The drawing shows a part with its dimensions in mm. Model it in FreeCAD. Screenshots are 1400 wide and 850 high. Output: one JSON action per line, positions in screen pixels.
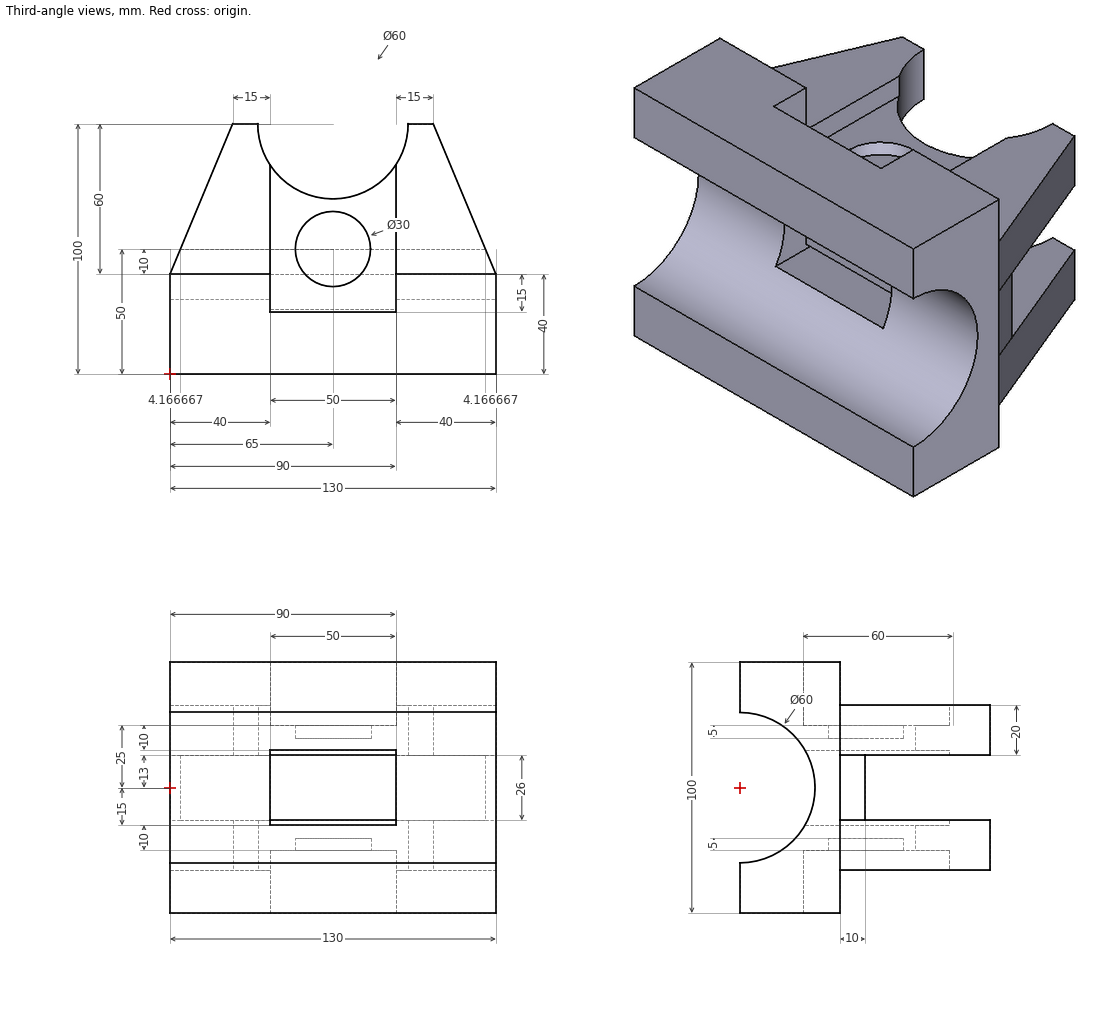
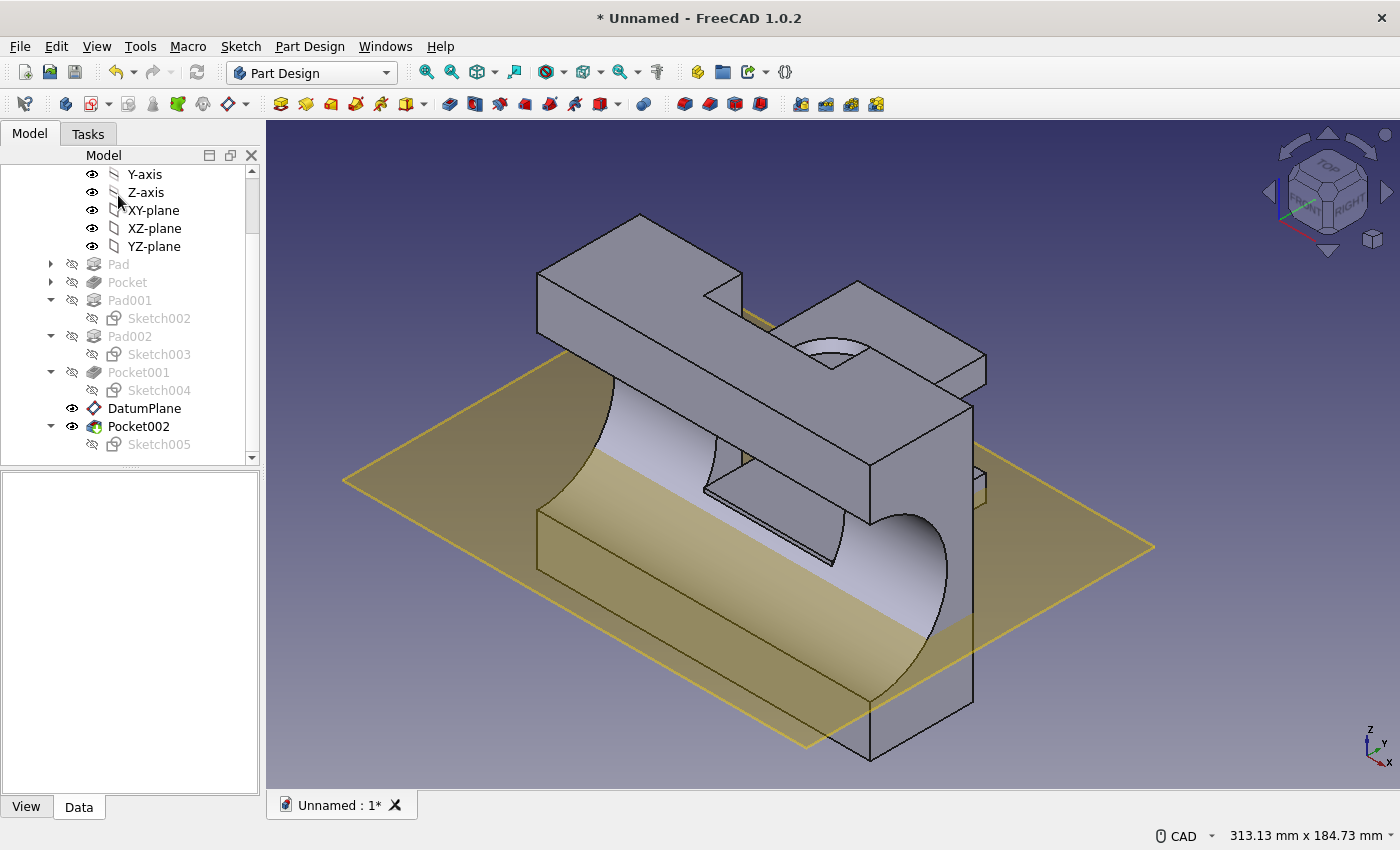
{"action": "left_click", "coordinate": [117, 408]}
{"action": "key", "text": "space"}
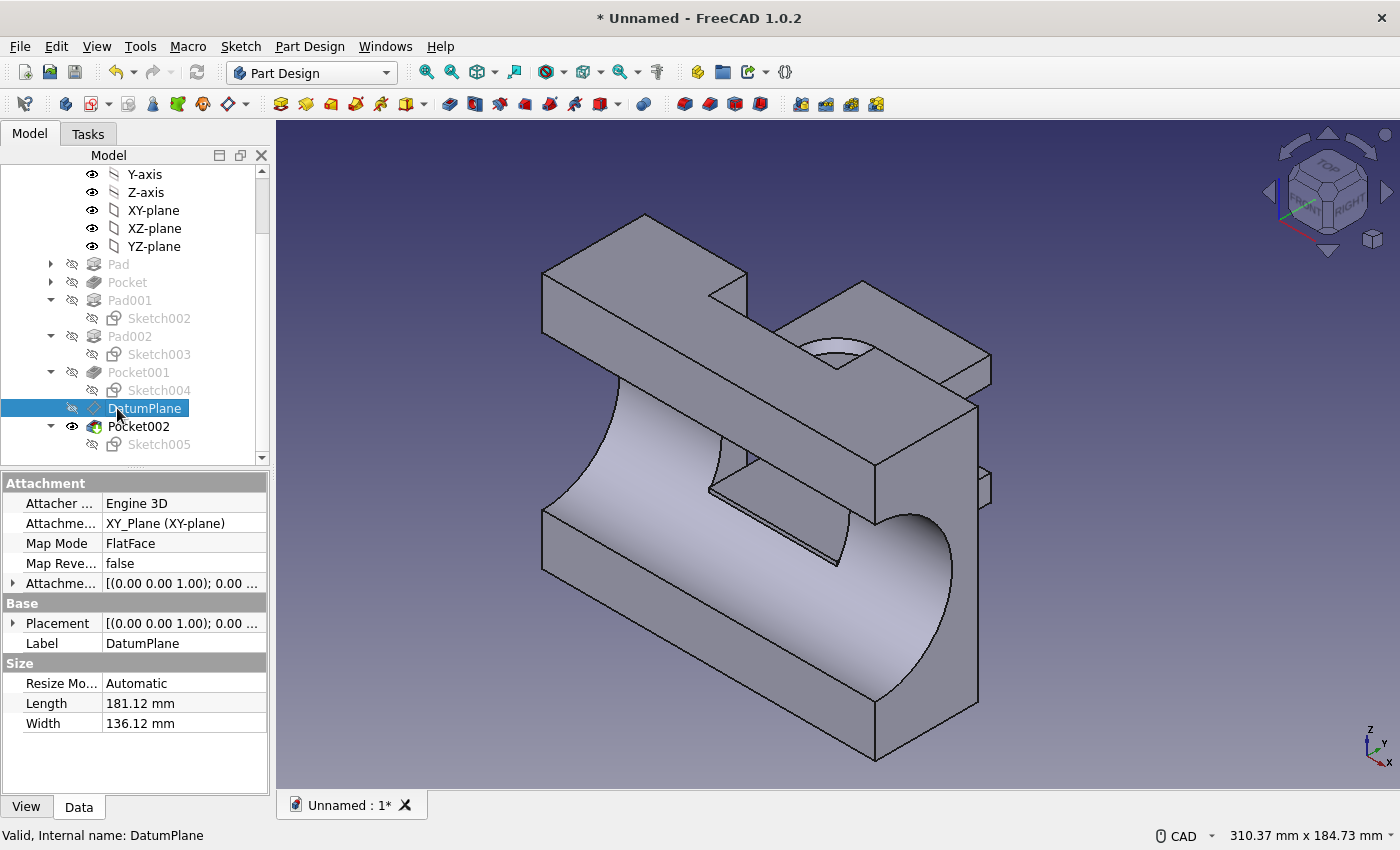
{"action": "scroll", "coordinate": [161, 314], "scroll_direction": "down", "scroll_amount": 3}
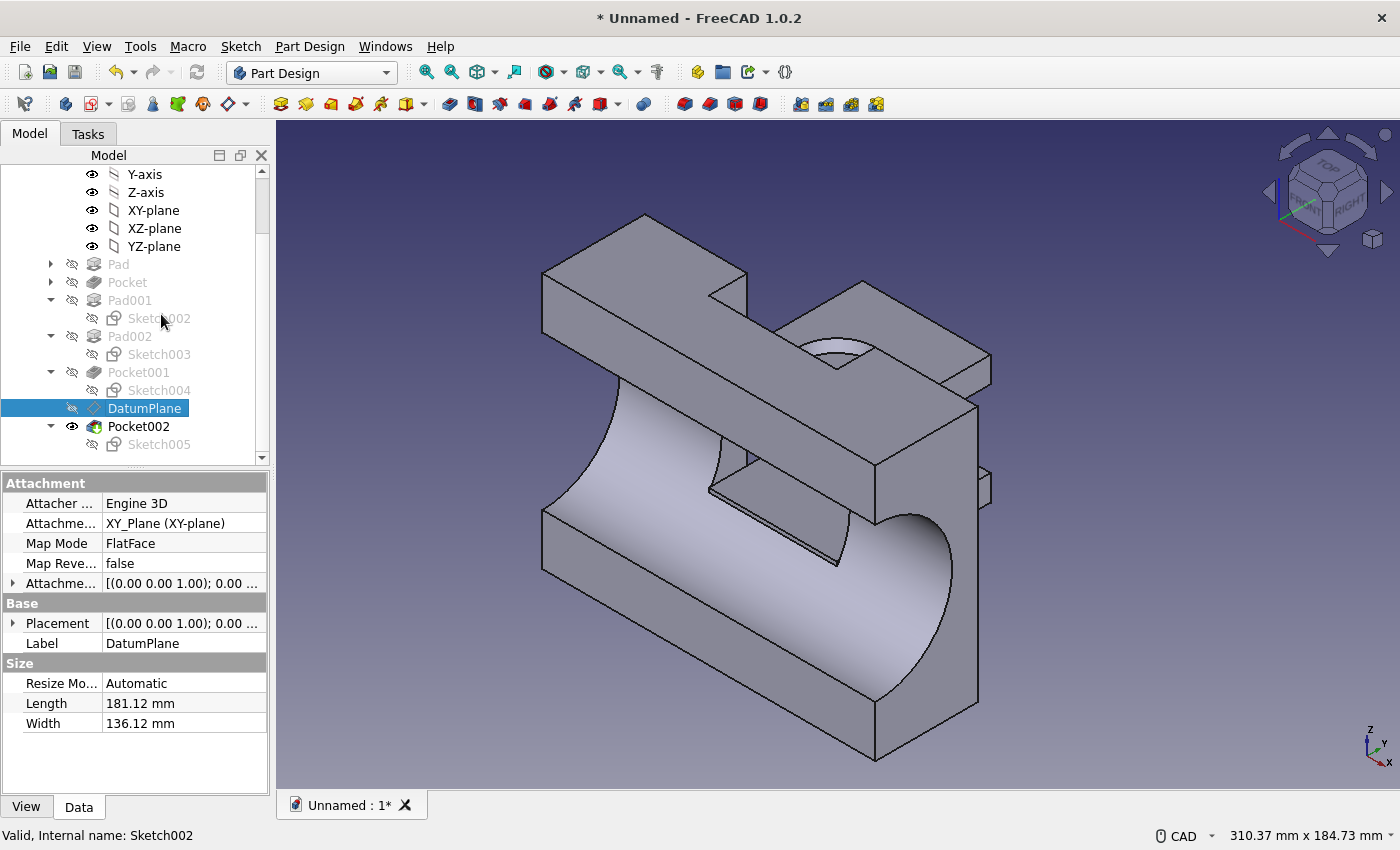
{"action": "scroll", "coordinate": [161, 314], "scroll_direction": "up", "scroll_amount": 15}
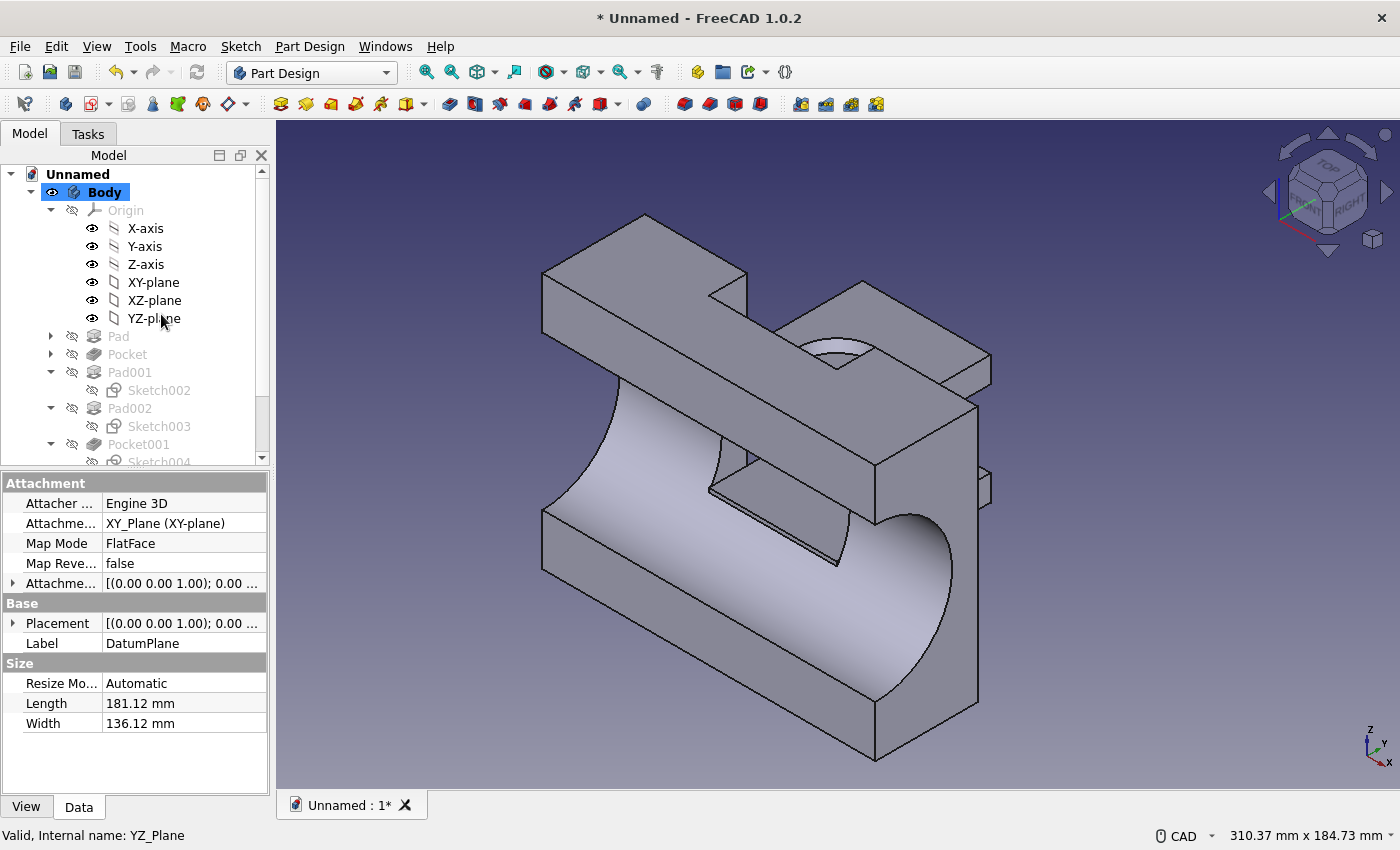
{"action": "left_click", "coordinate": [137, 282]}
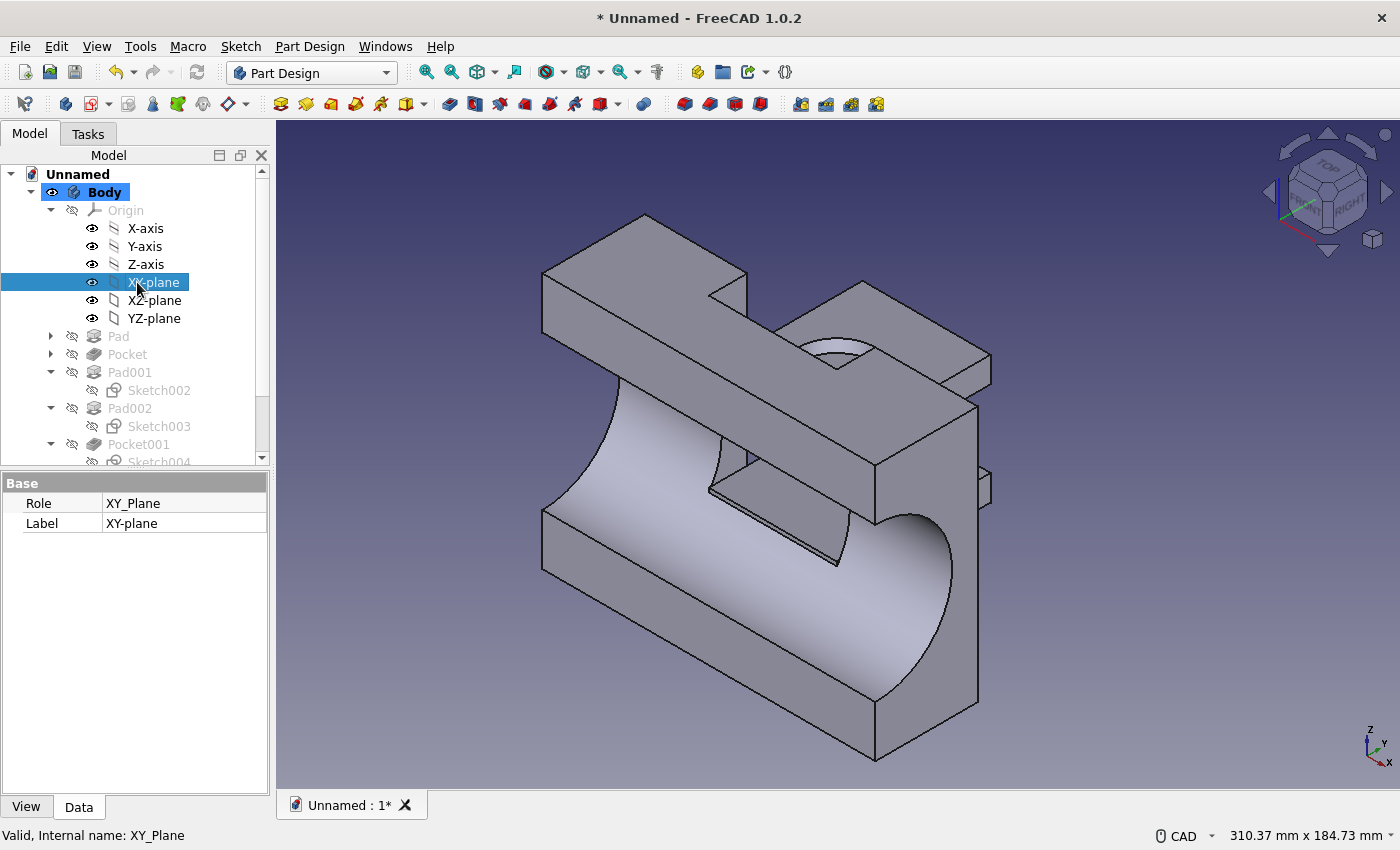
{"action": "left_click", "coordinate": [228, 104]}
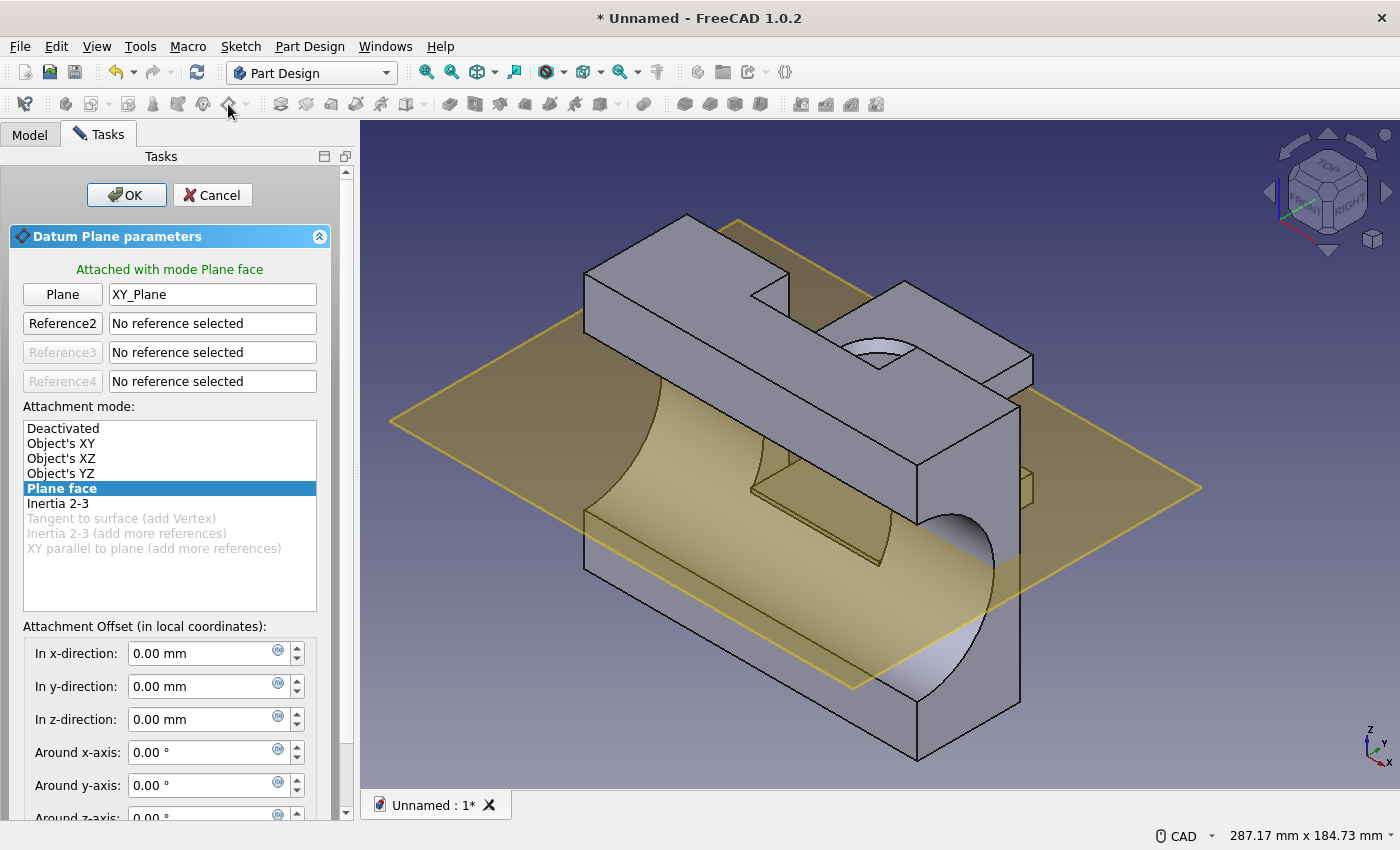
{"action": "triple_click", "coordinate": [210, 720]}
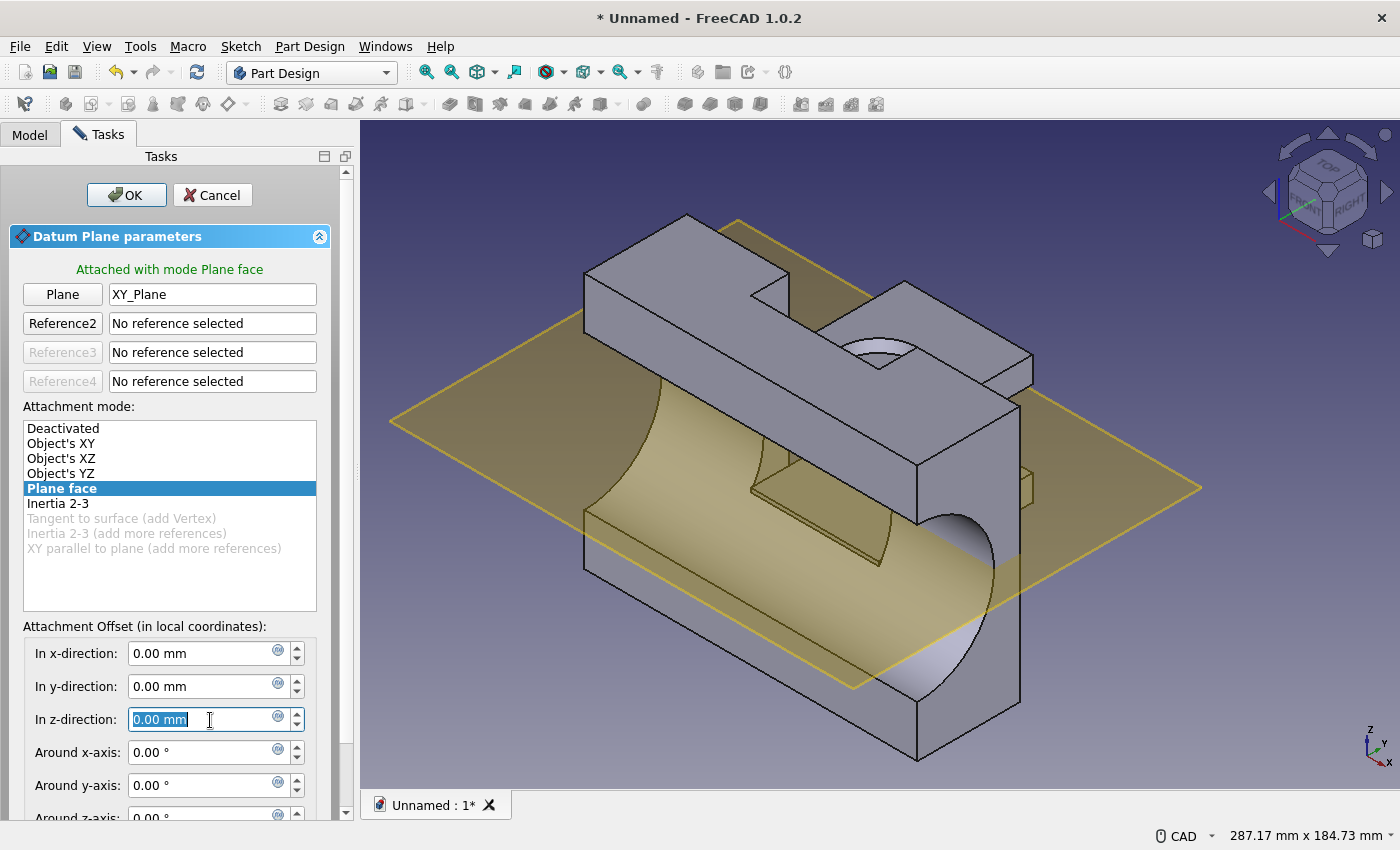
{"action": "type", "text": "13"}
{"action": "key", "text": "Tab"}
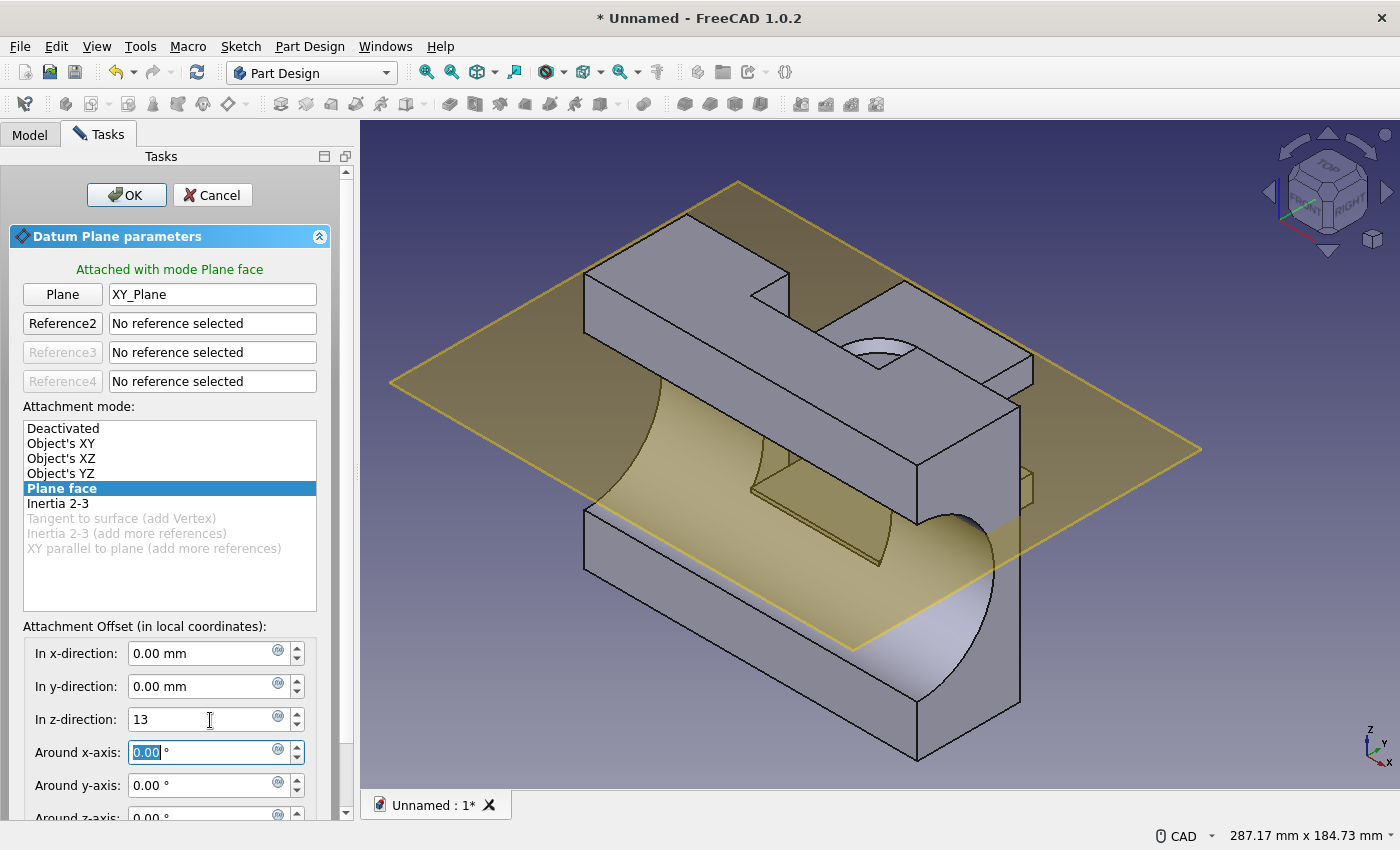
{"action": "left_click", "coordinate": [127, 195]}